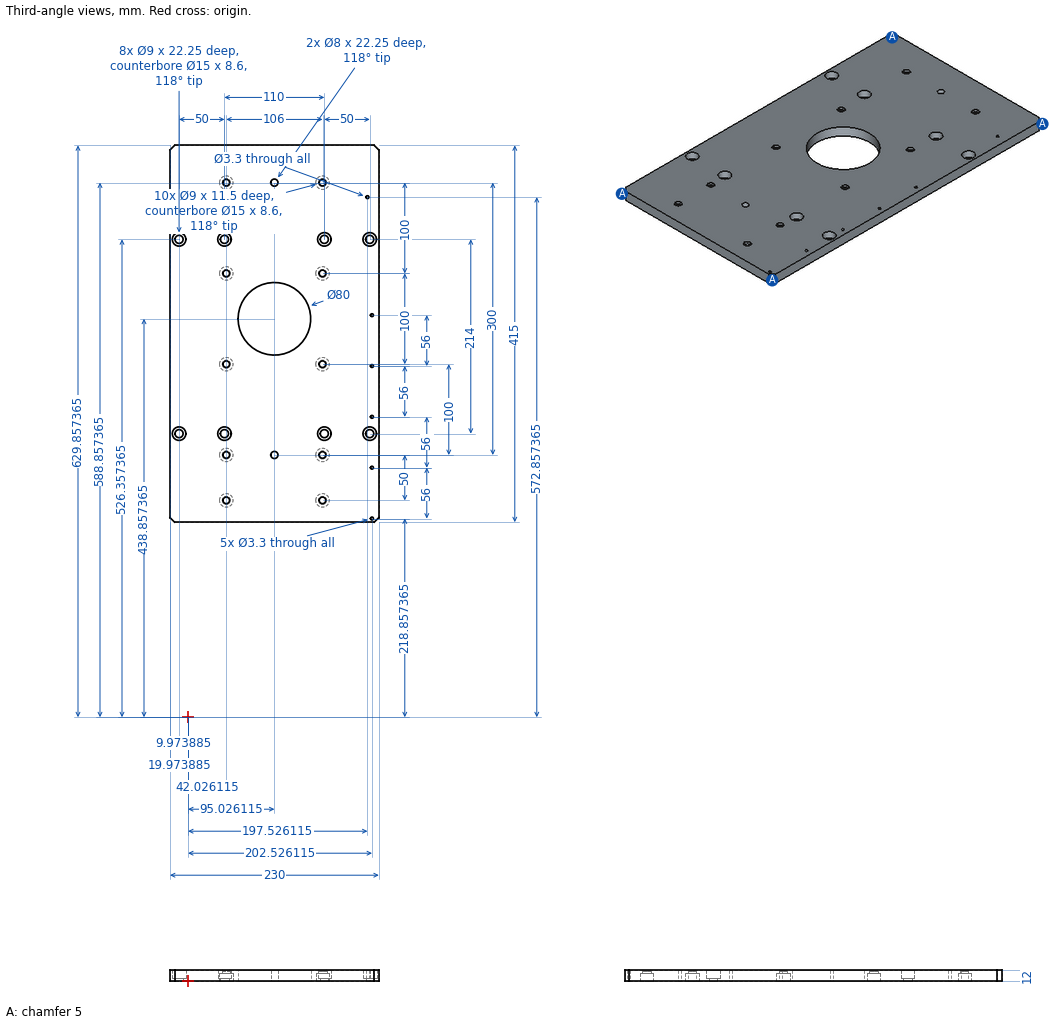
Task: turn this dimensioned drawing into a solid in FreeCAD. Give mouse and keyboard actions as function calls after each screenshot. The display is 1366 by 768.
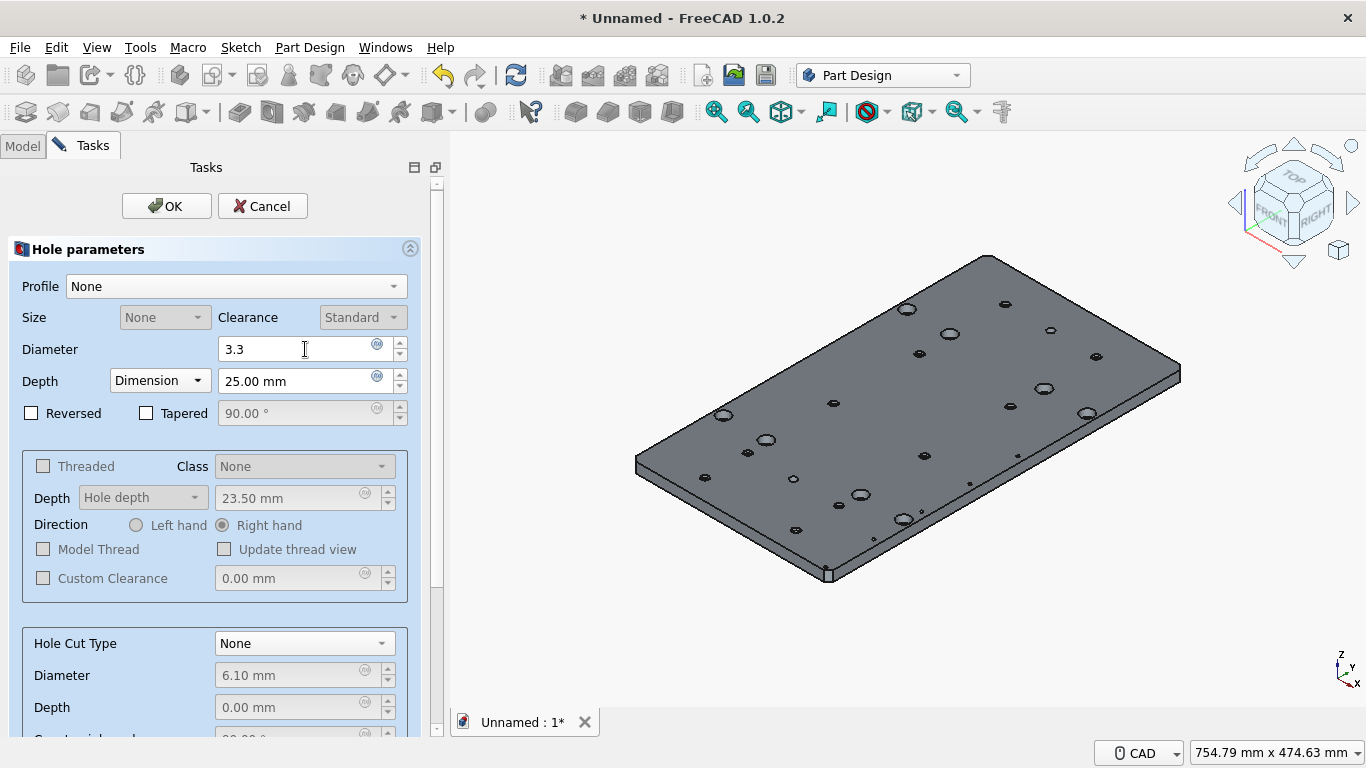
click(161, 380)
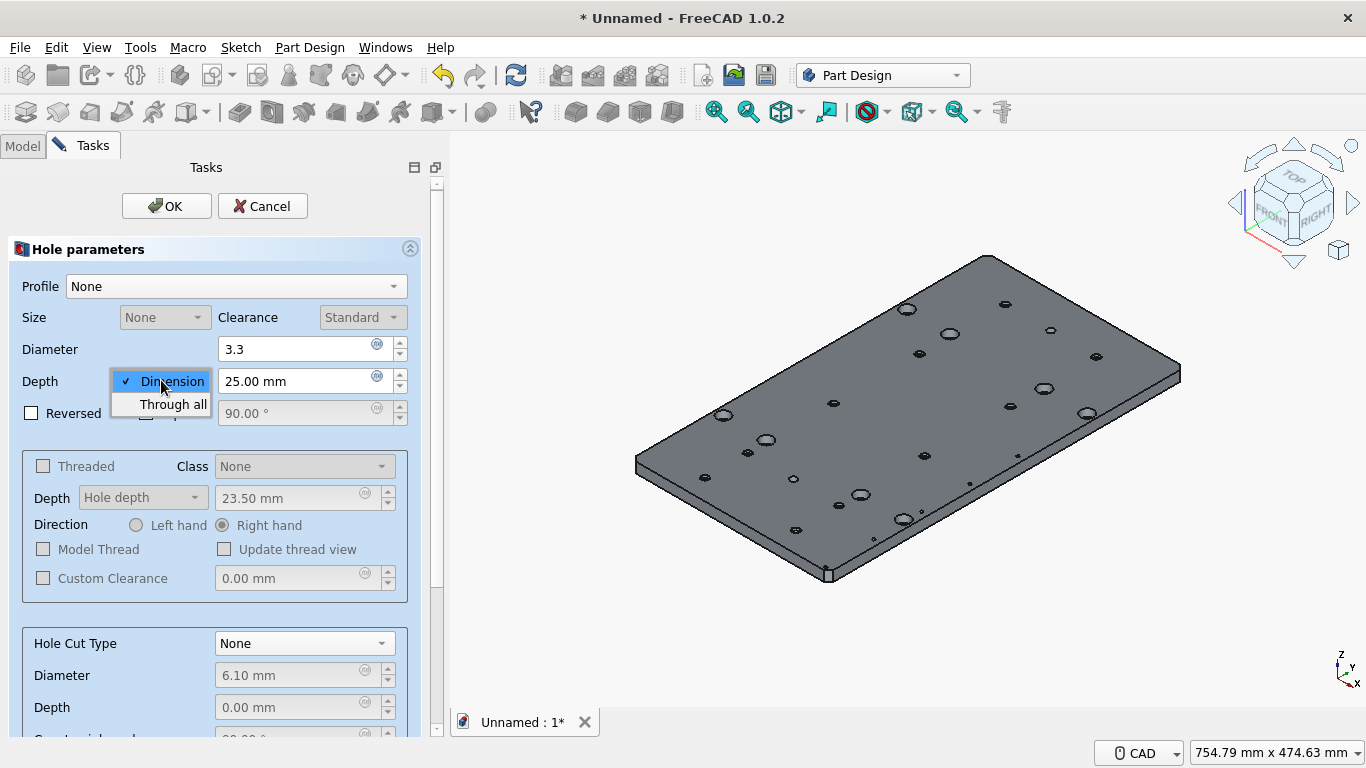
click(160, 404)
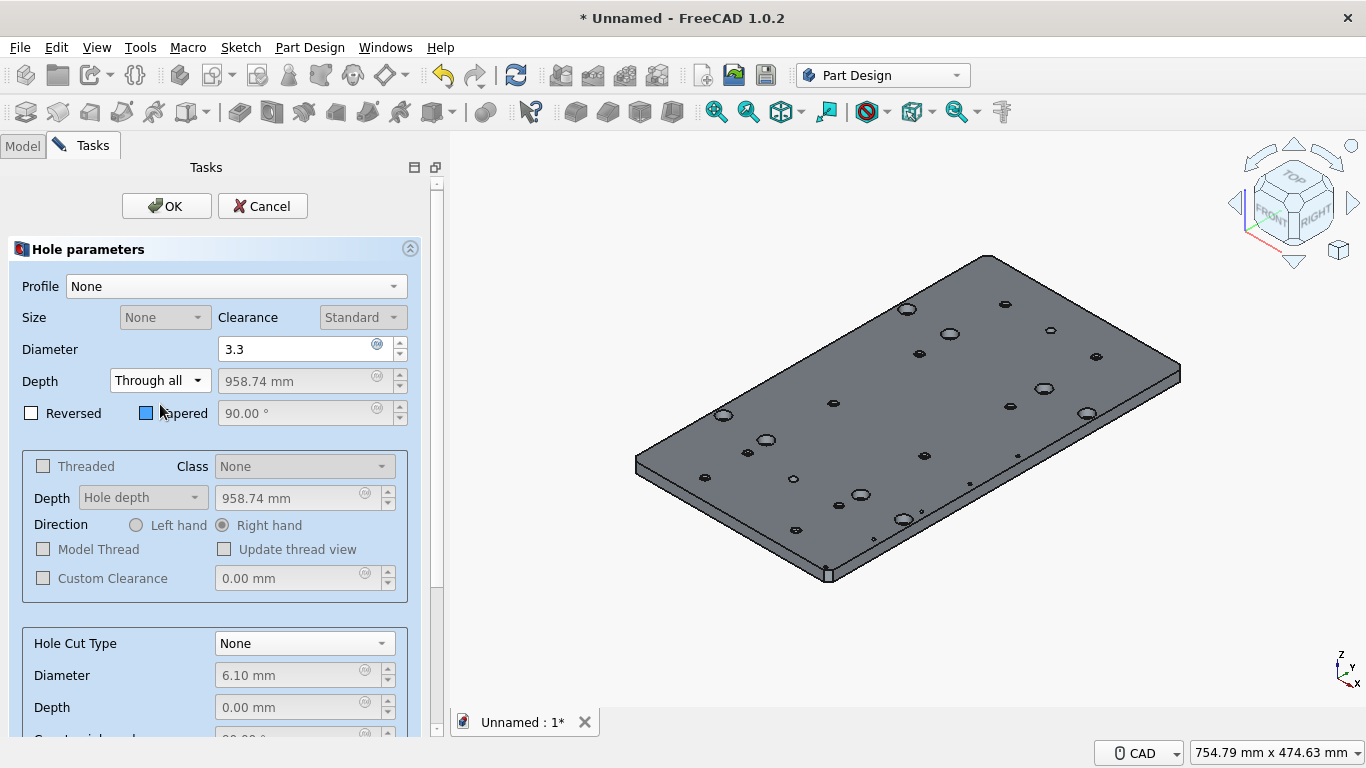
click(167, 206)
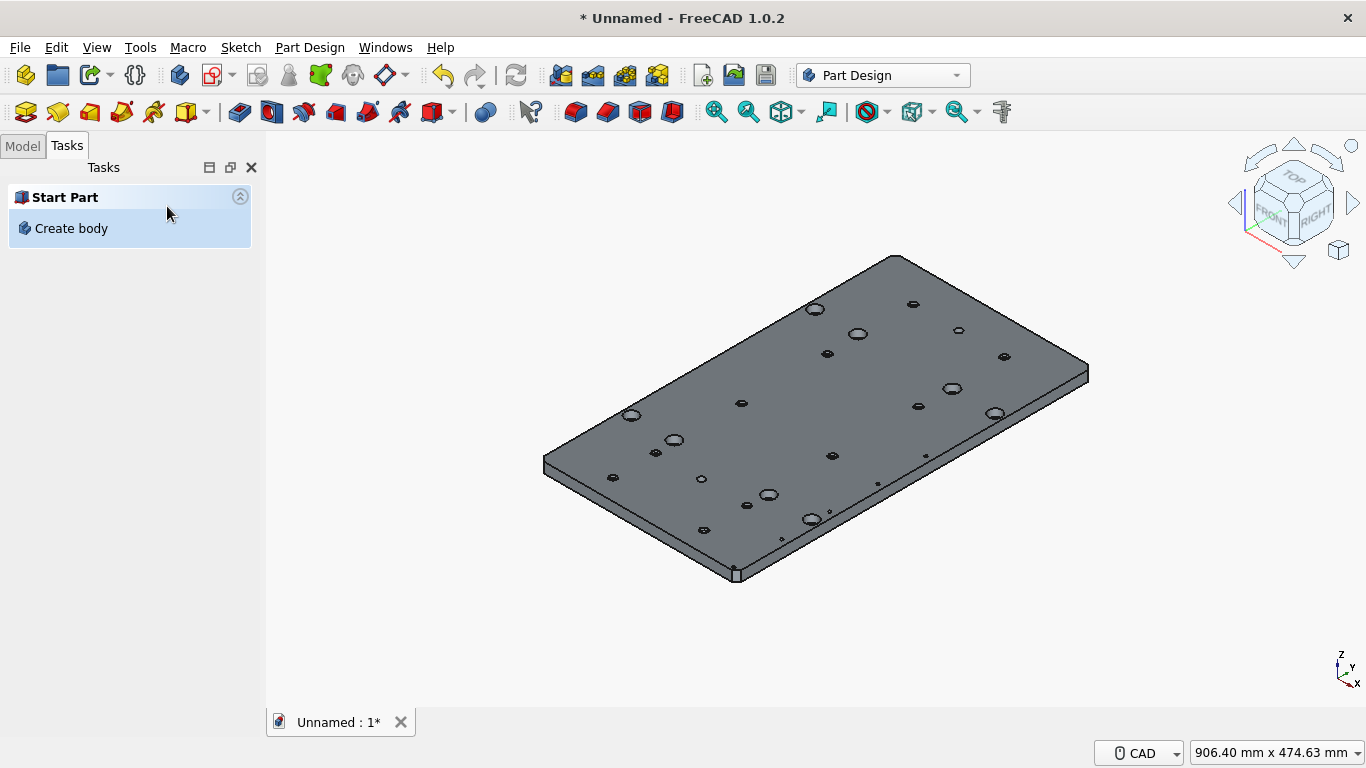
click(816, 412)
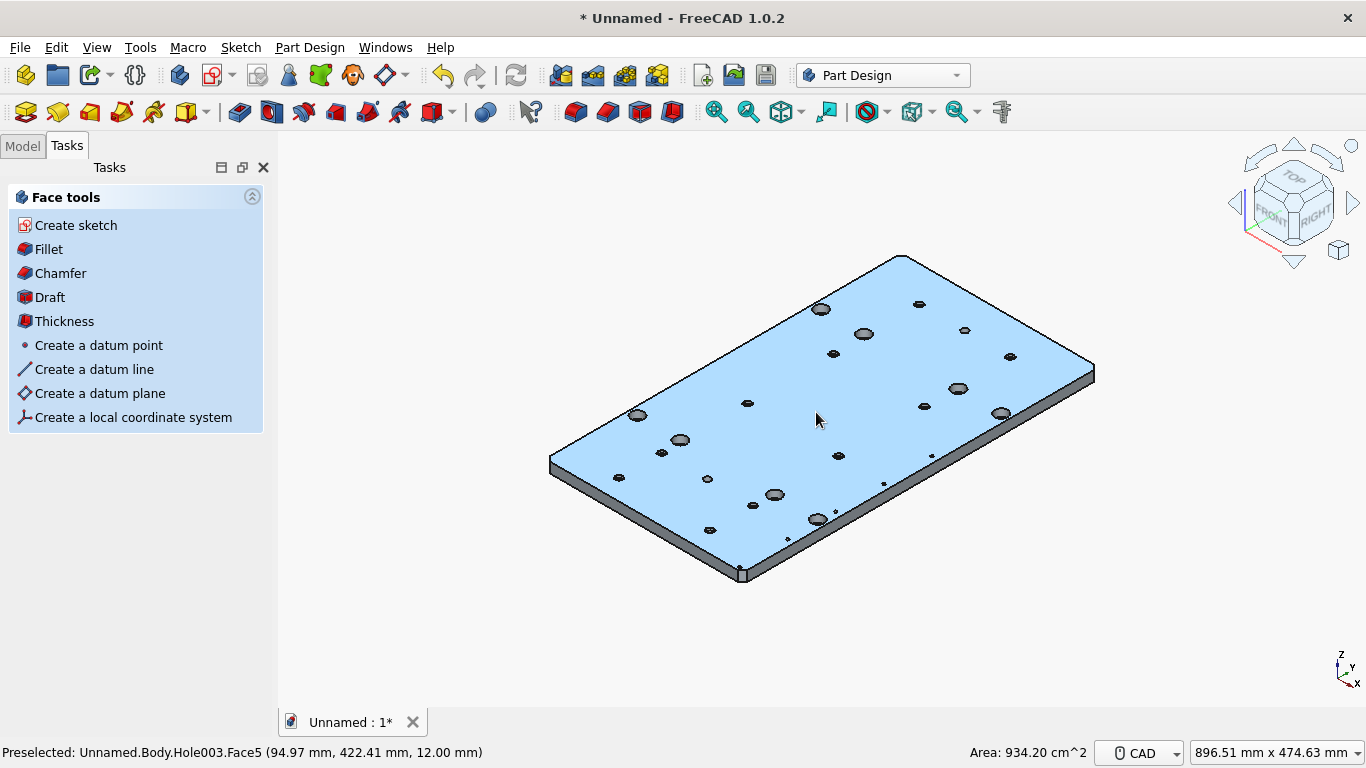
click(212, 76)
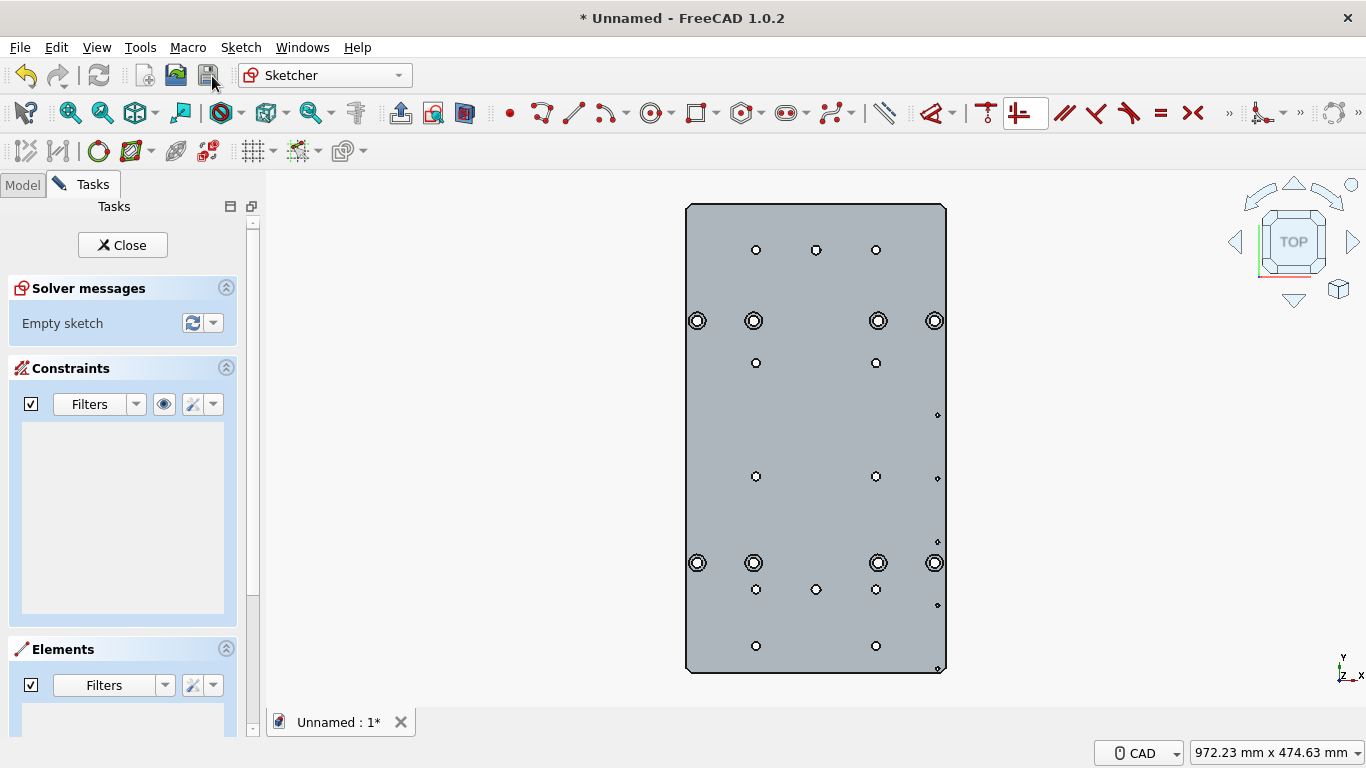
scroll(942, 259, up, 15)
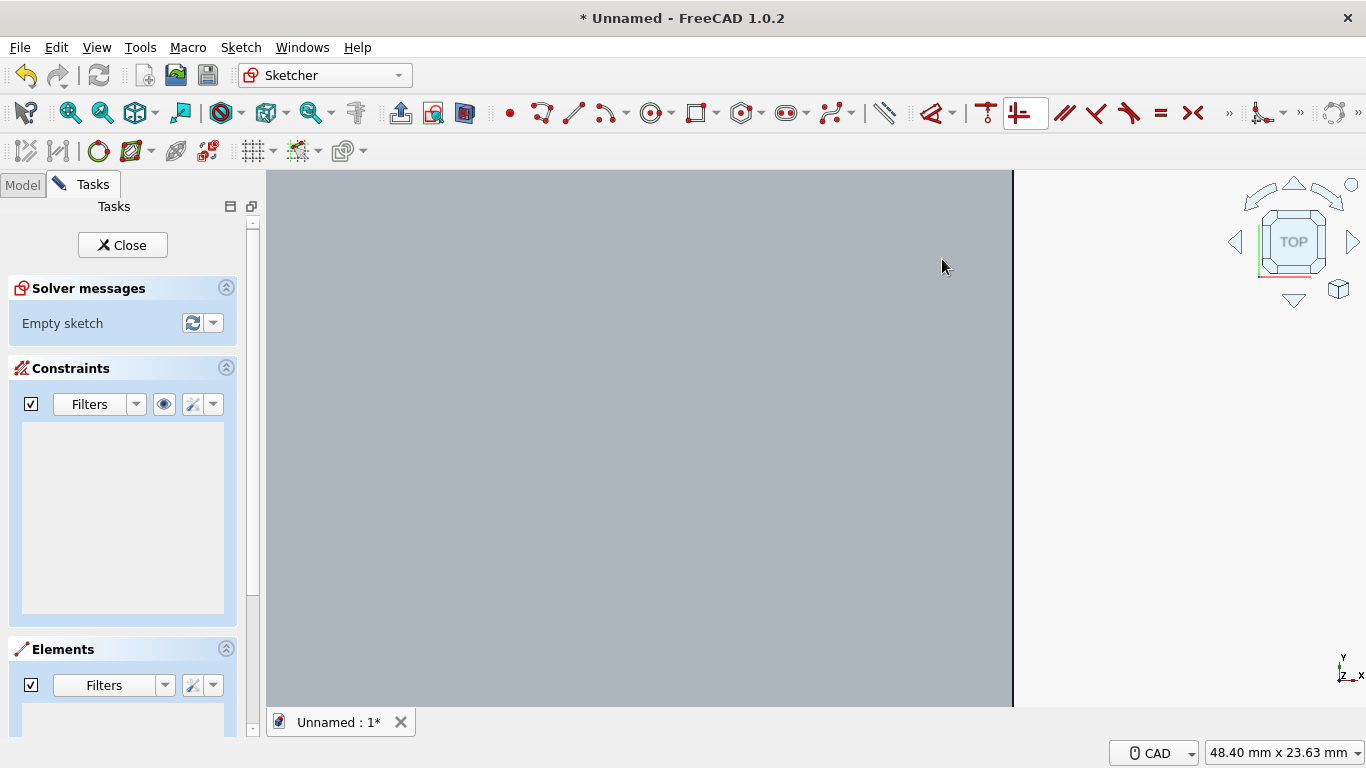
scroll(724, 442, up, 8)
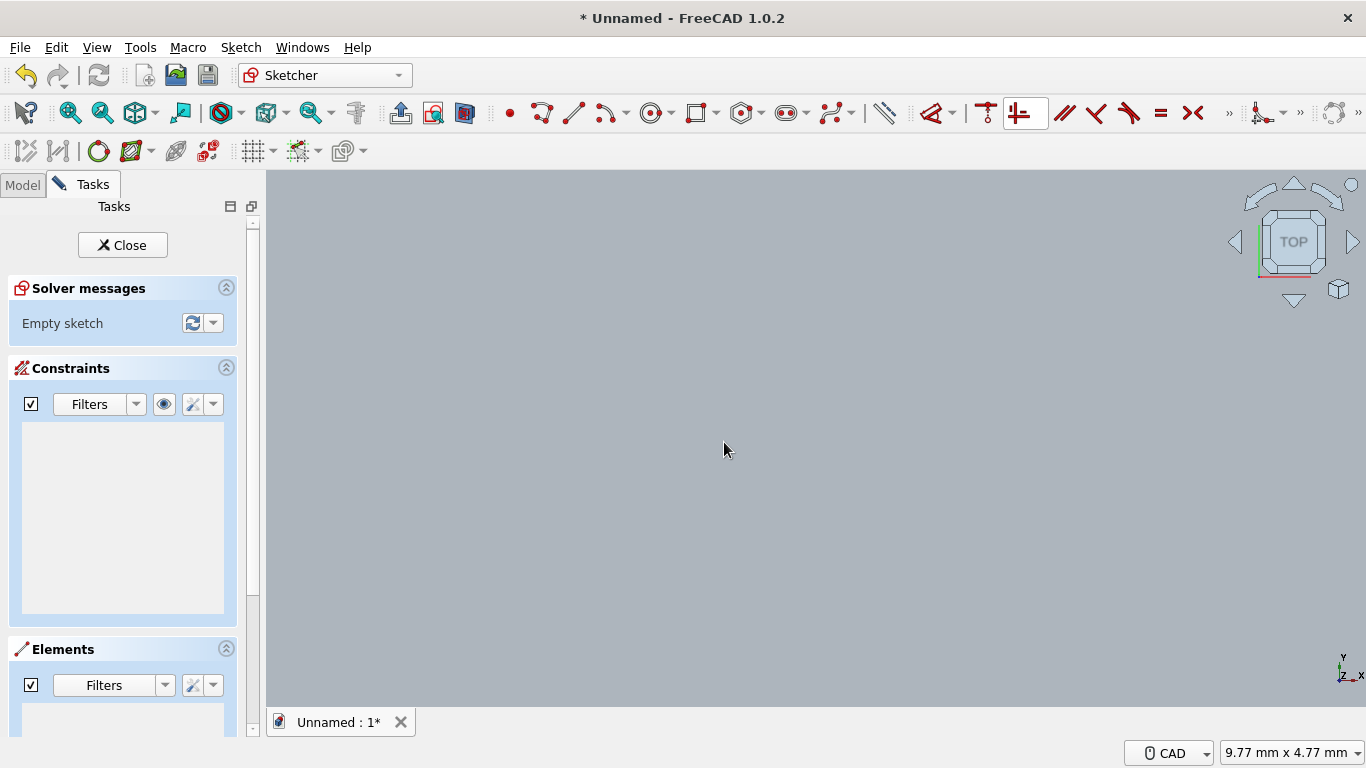
click(652, 114)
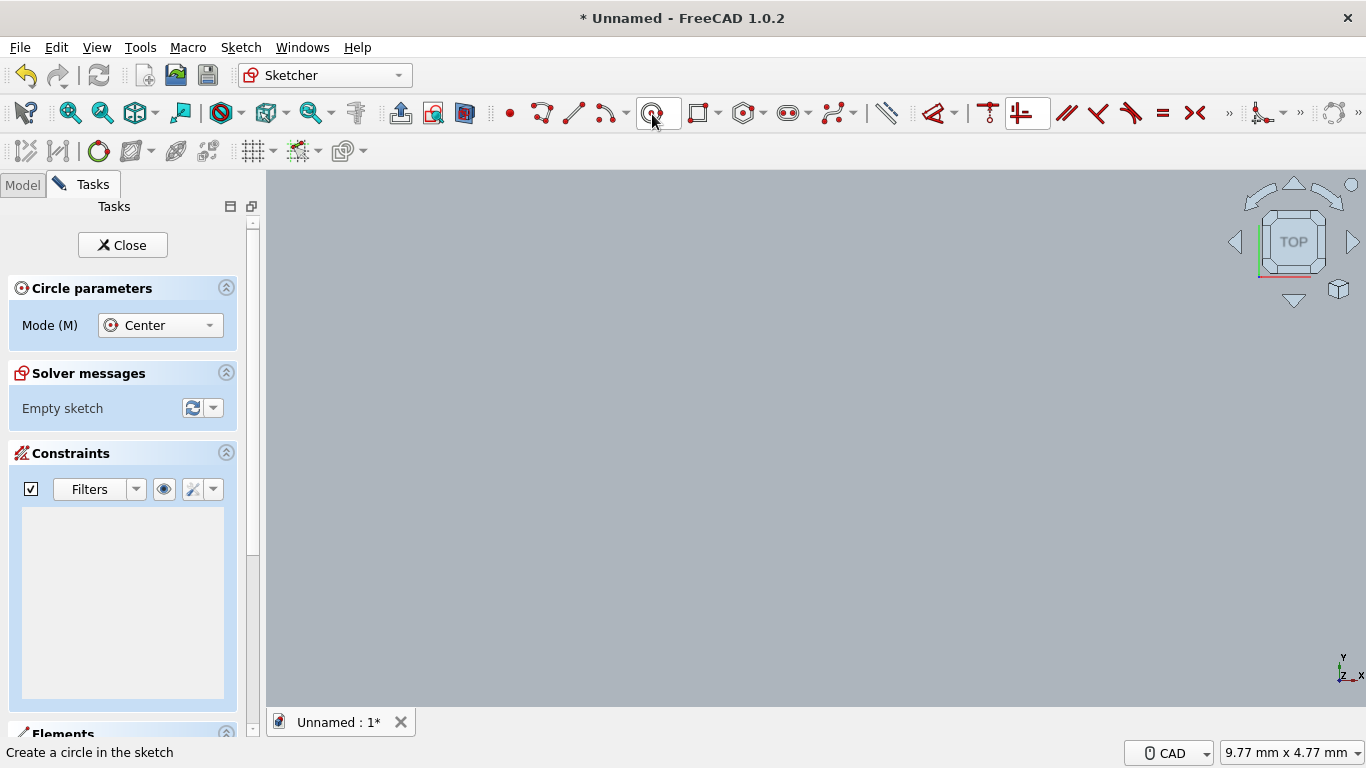
click(746, 435)
move(878, 304)